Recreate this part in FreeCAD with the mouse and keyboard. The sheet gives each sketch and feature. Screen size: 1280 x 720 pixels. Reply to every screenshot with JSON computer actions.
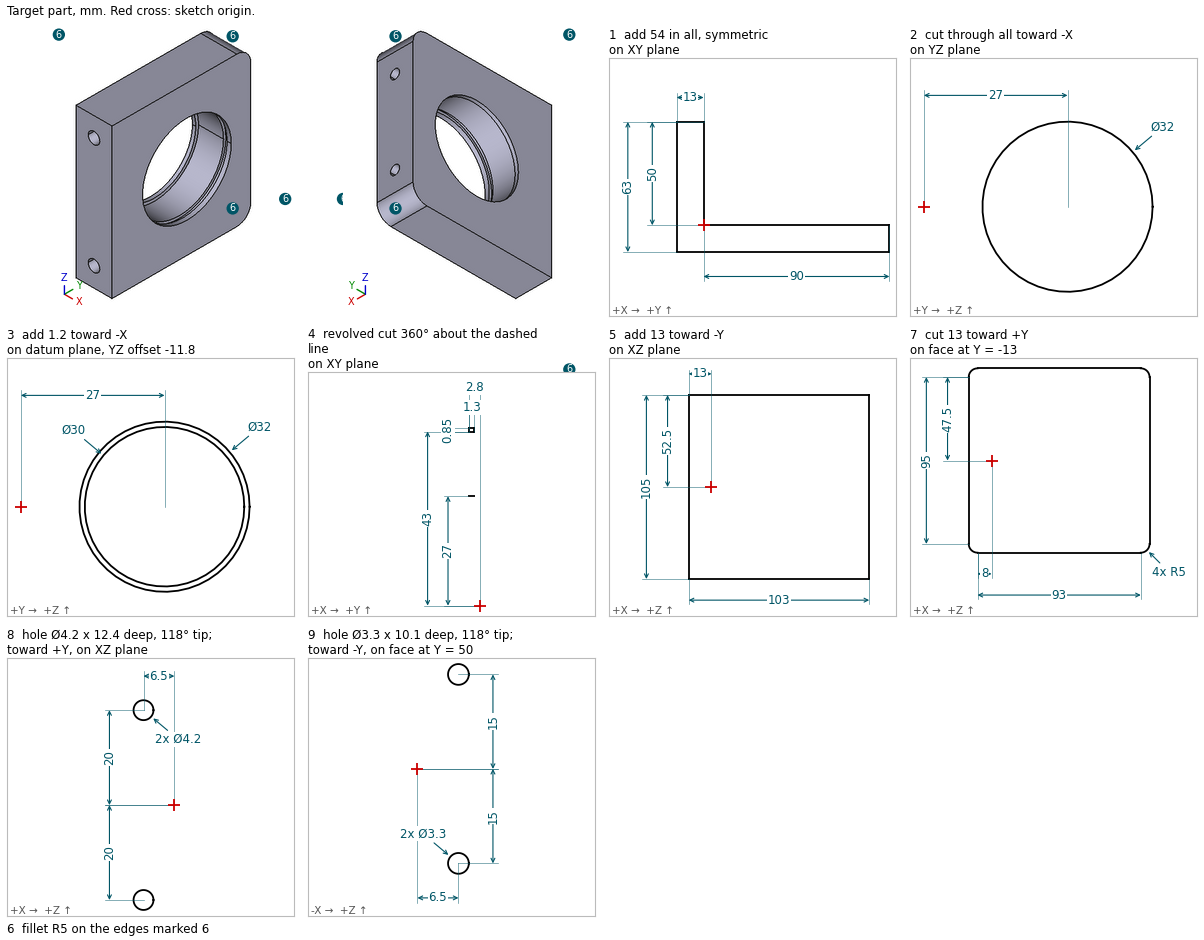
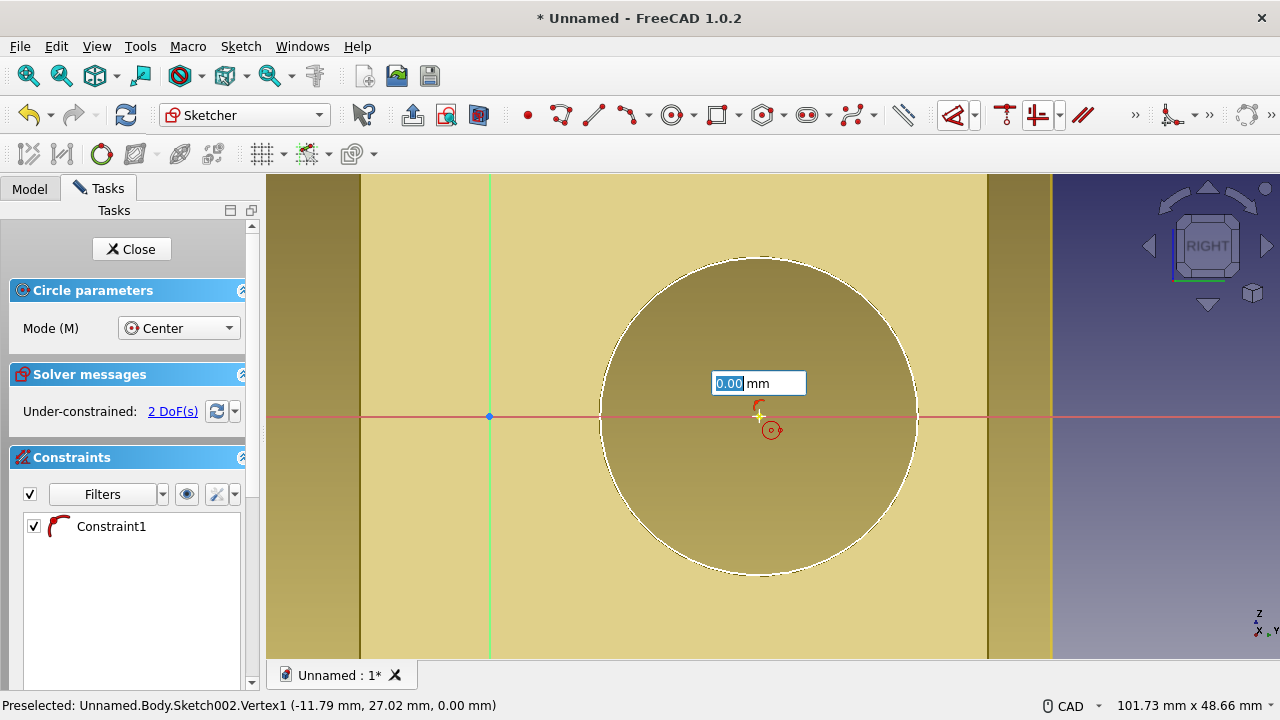
{"action": "scroll", "coordinate": [899, 365], "scroll_direction": "up", "scroll_amount": 3}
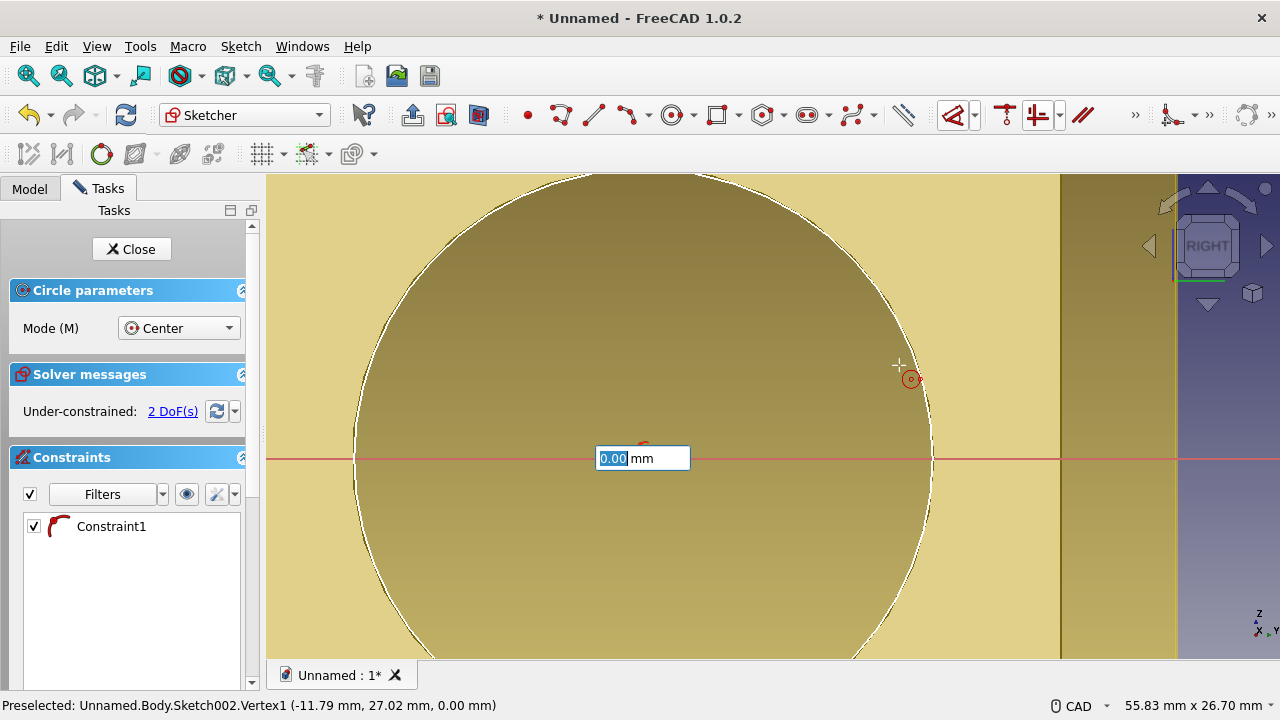
{"action": "left_click", "coordinate": [899, 365]}
{"action": "key", "text": "Escape"}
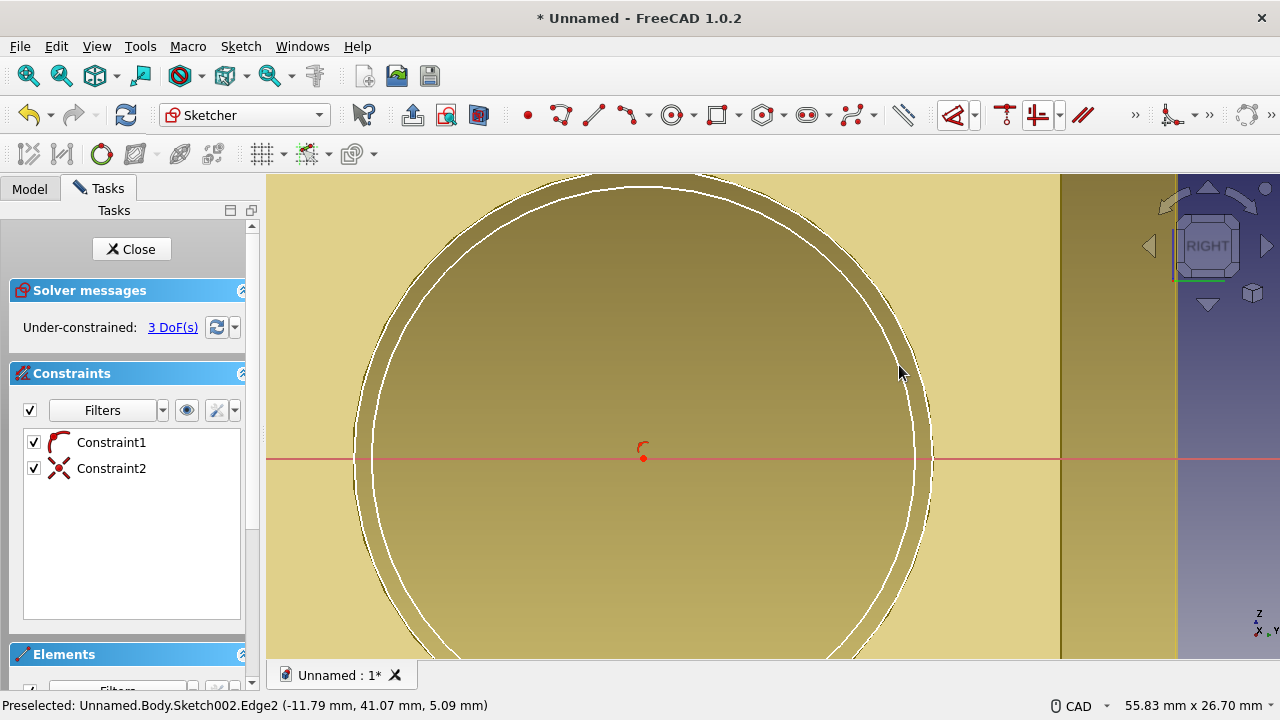
{"action": "left_click", "coordinate": [847, 253]}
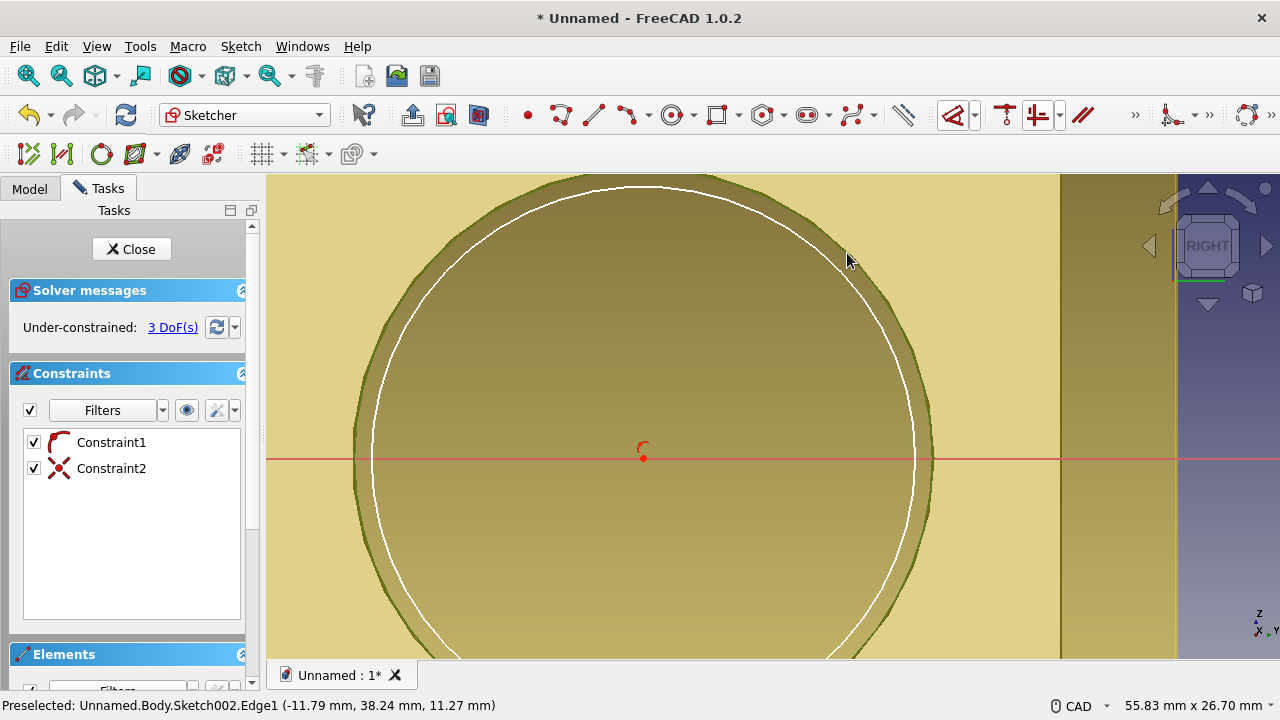
{"action": "left_click", "coordinate": [974, 116]}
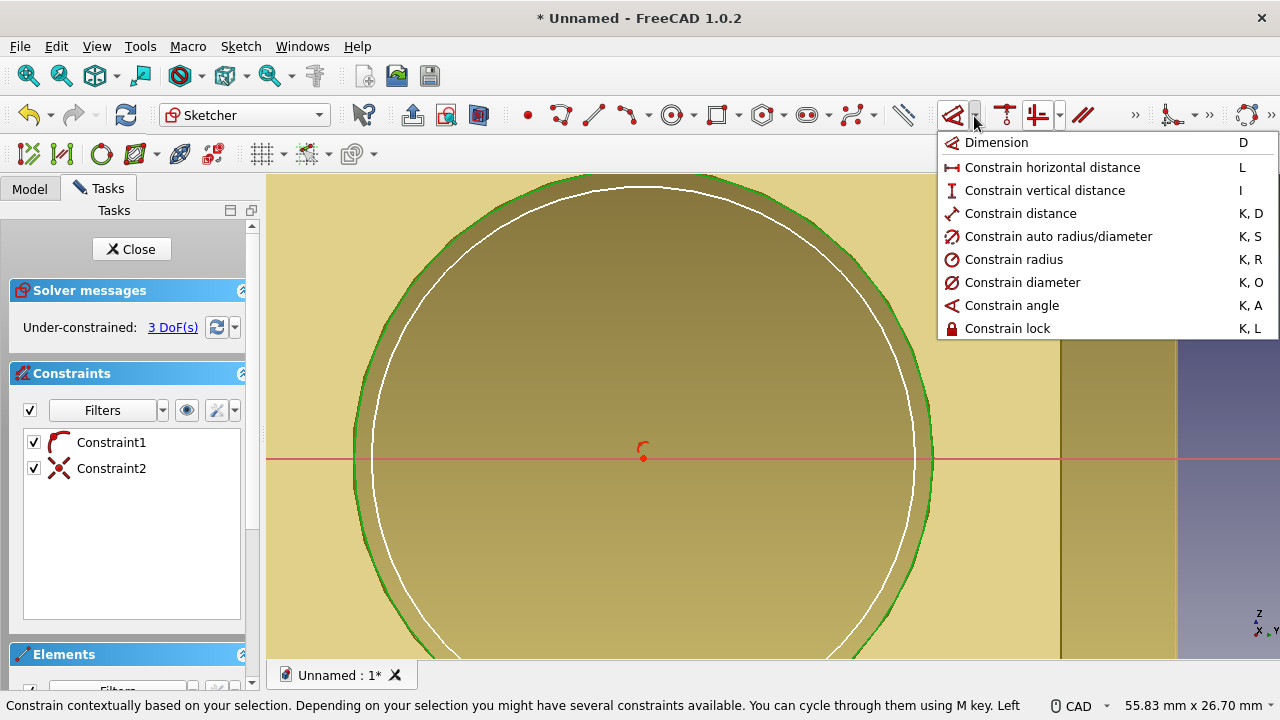
{"action": "left_click", "coordinate": [1108, 282]}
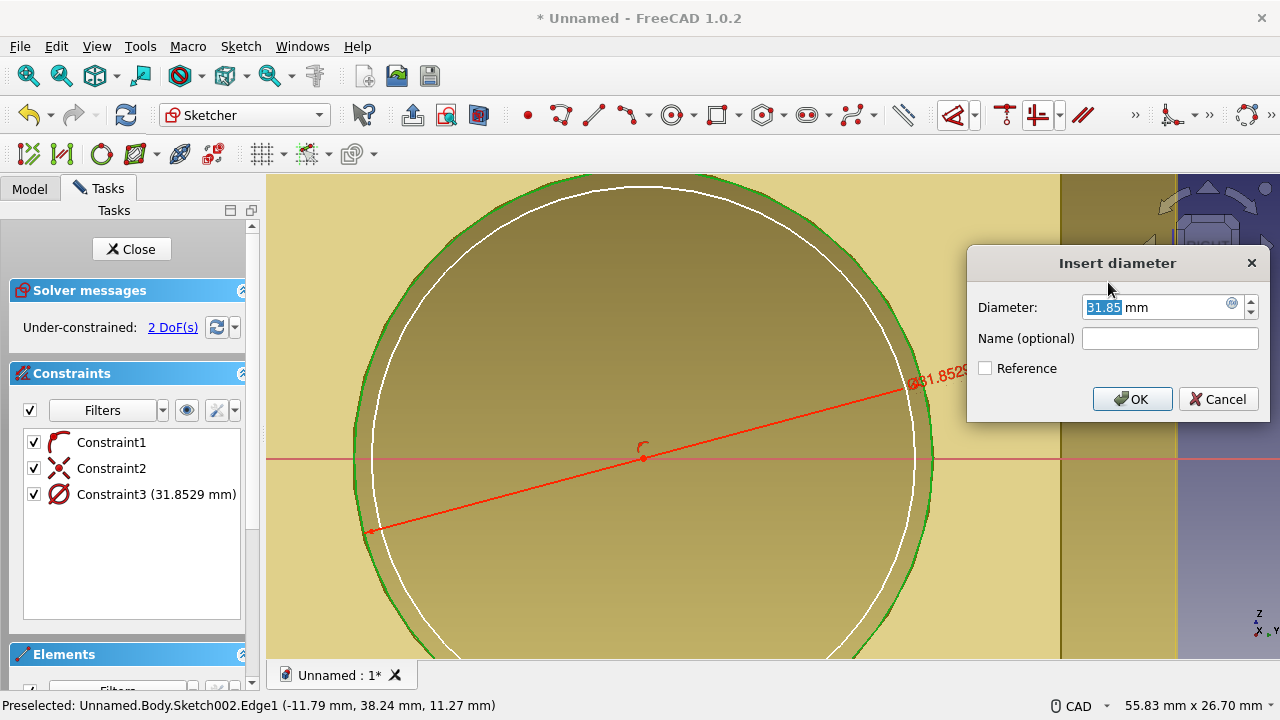
{"action": "type", "text": "32"}
{"action": "key", "text": "Return"}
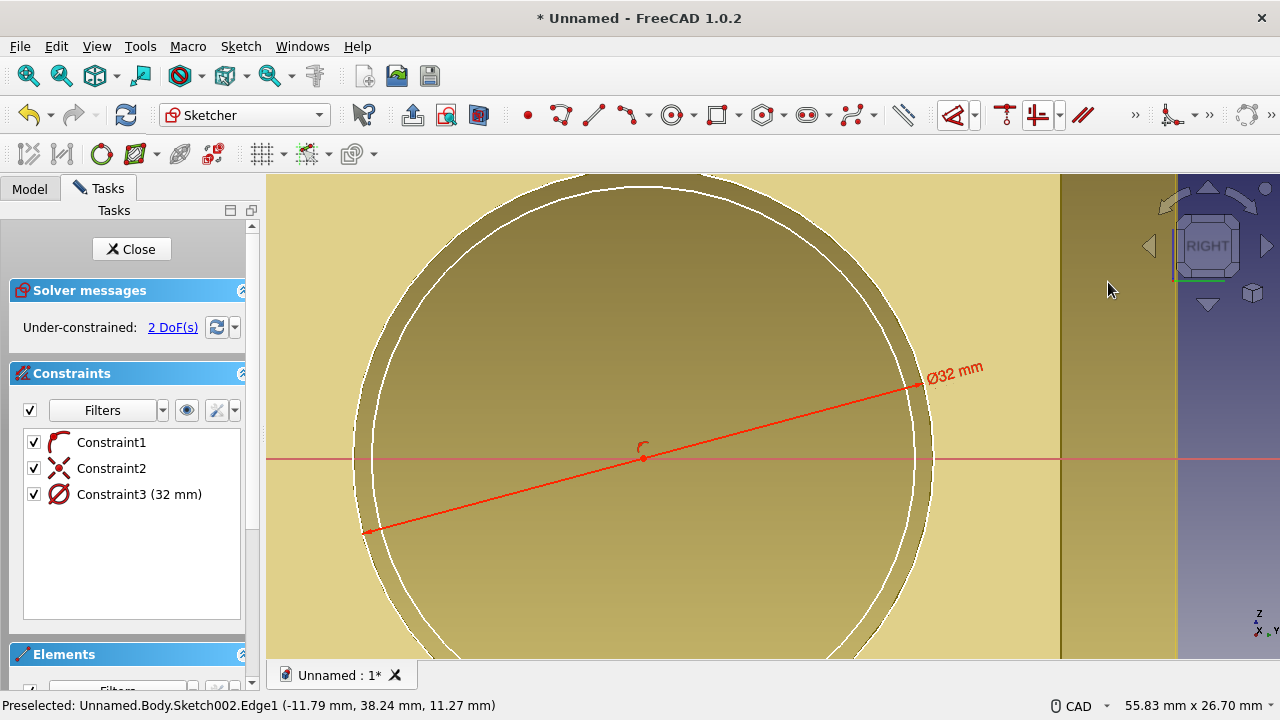
{"action": "left_click", "coordinate": [835, 266]}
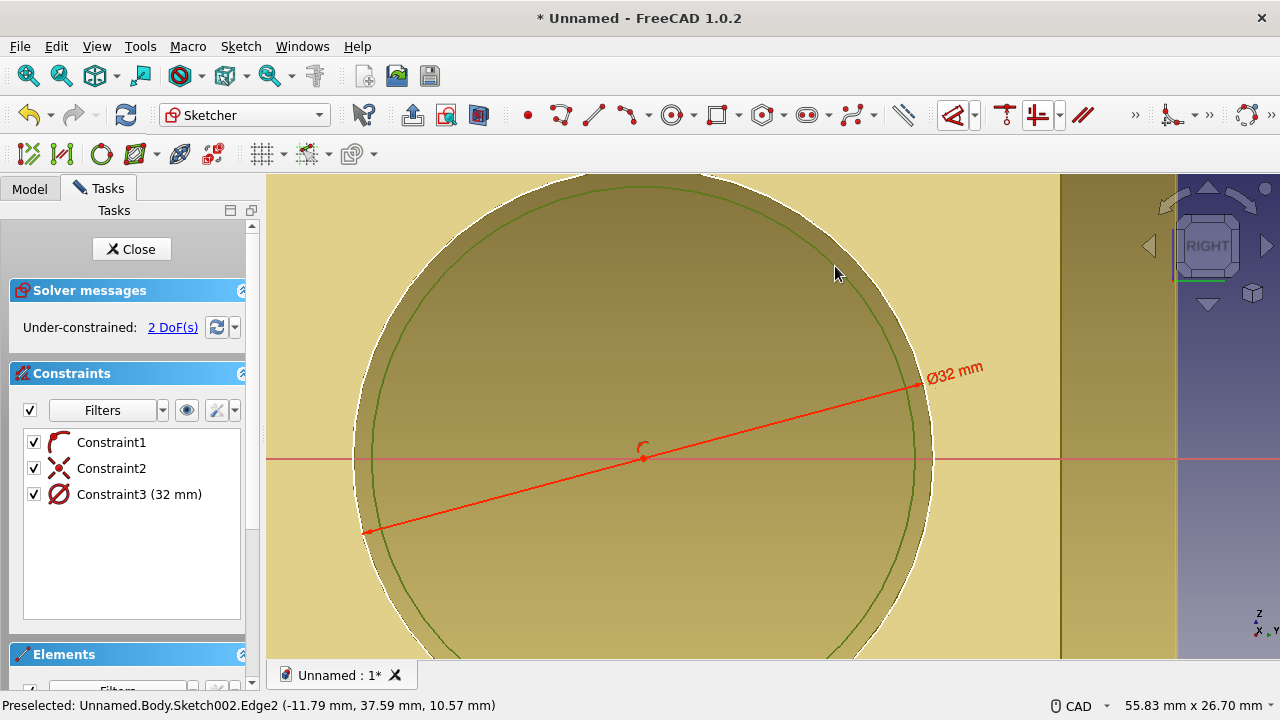
{"action": "left_click", "coordinate": [974, 116]}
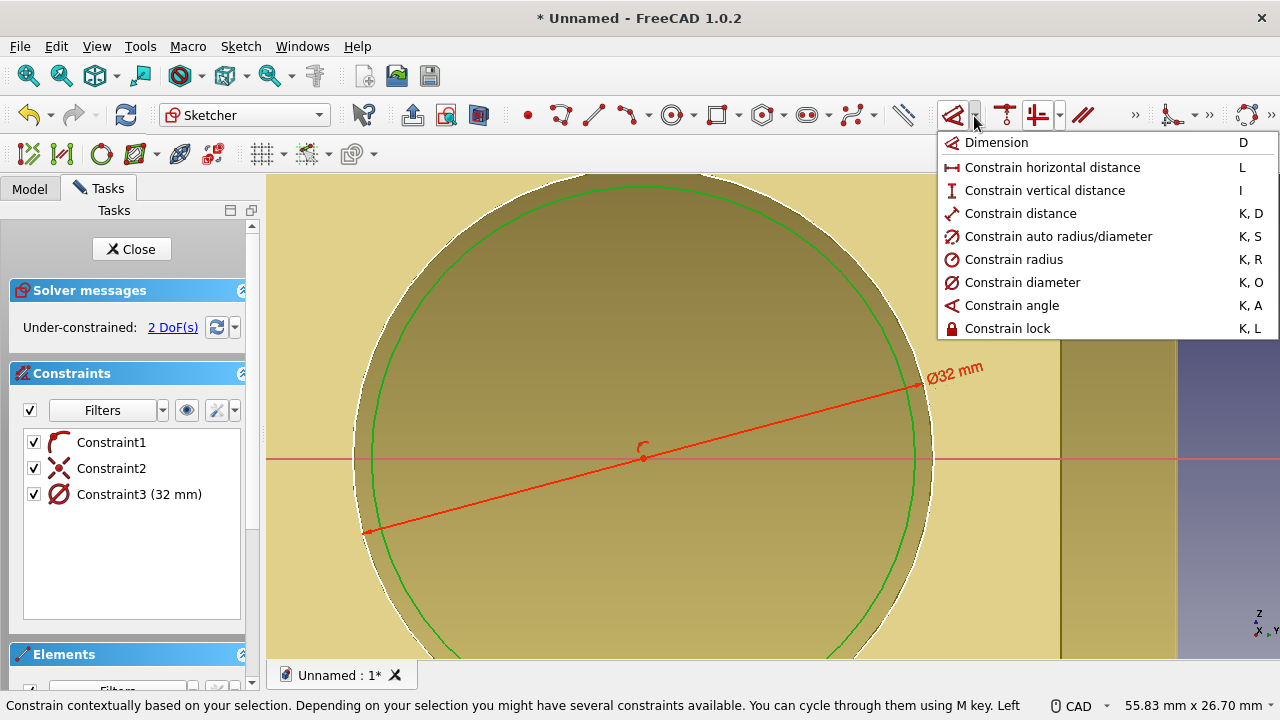
{"action": "left_click", "coordinate": [1108, 282]}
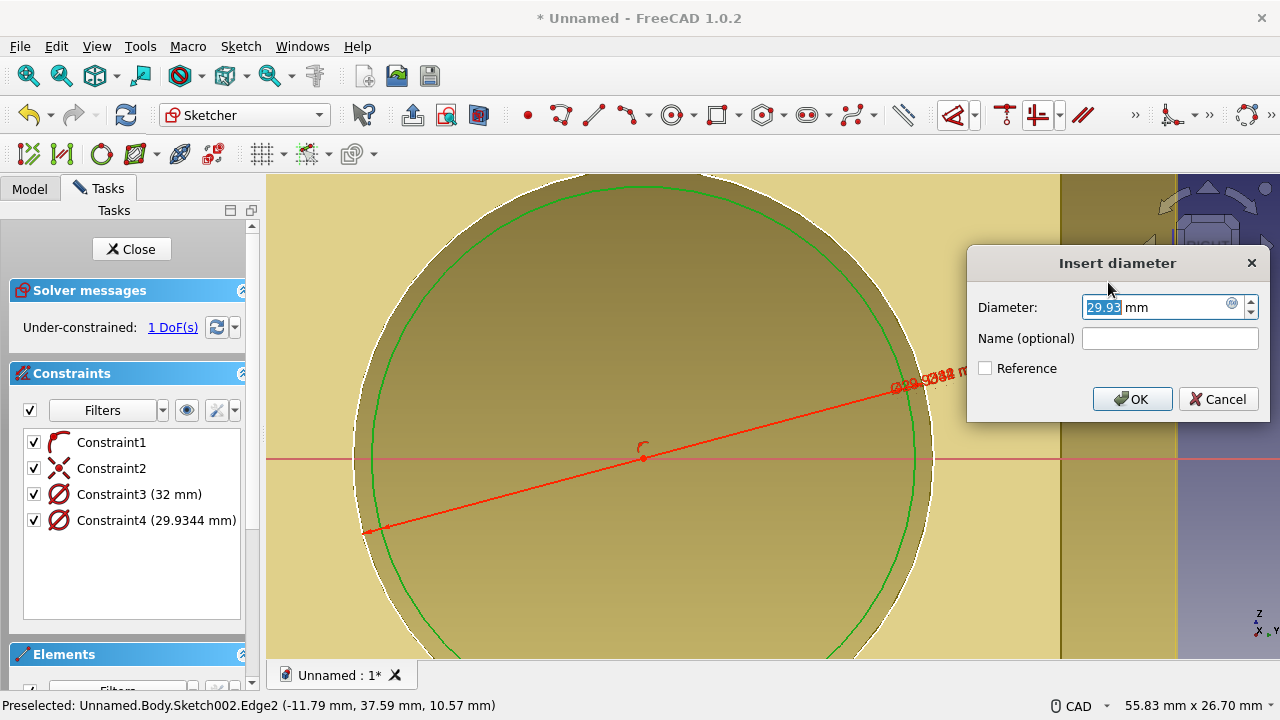
{"action": "type", "text": "30"}
{"action": "key", "text": "Return"}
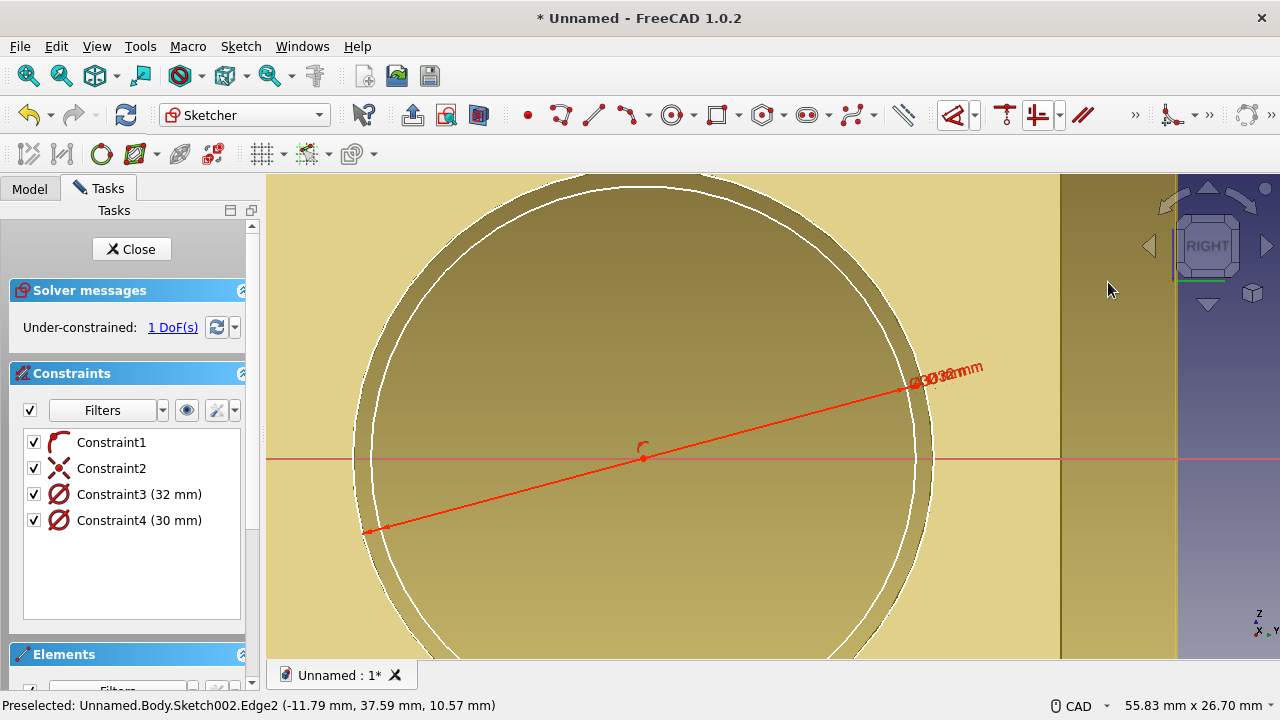
{"action": "left_click", "coordinate": [643, 459]}